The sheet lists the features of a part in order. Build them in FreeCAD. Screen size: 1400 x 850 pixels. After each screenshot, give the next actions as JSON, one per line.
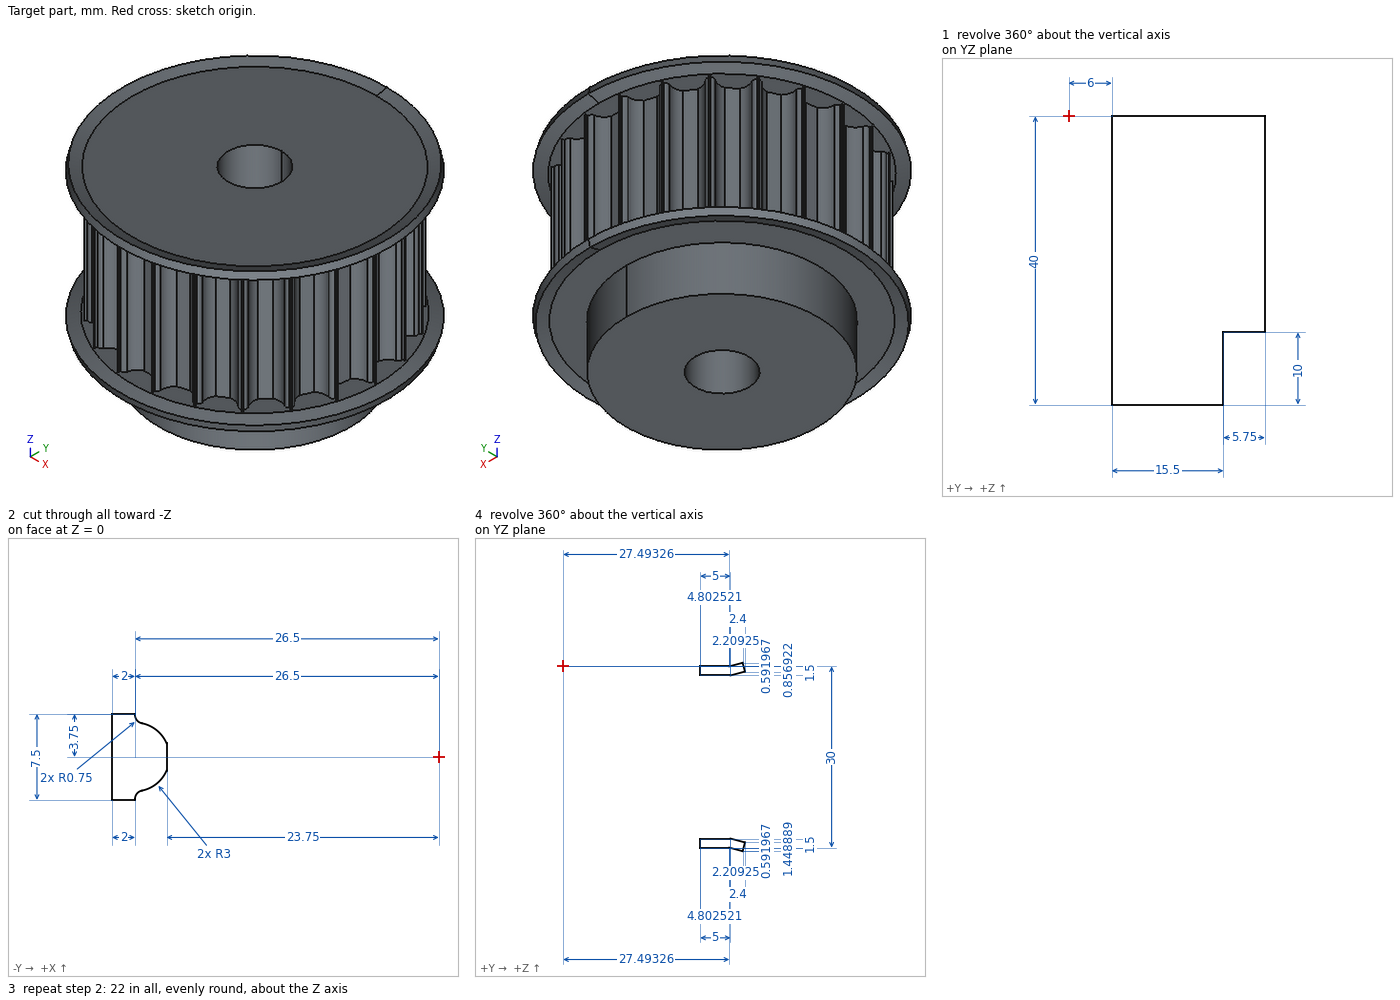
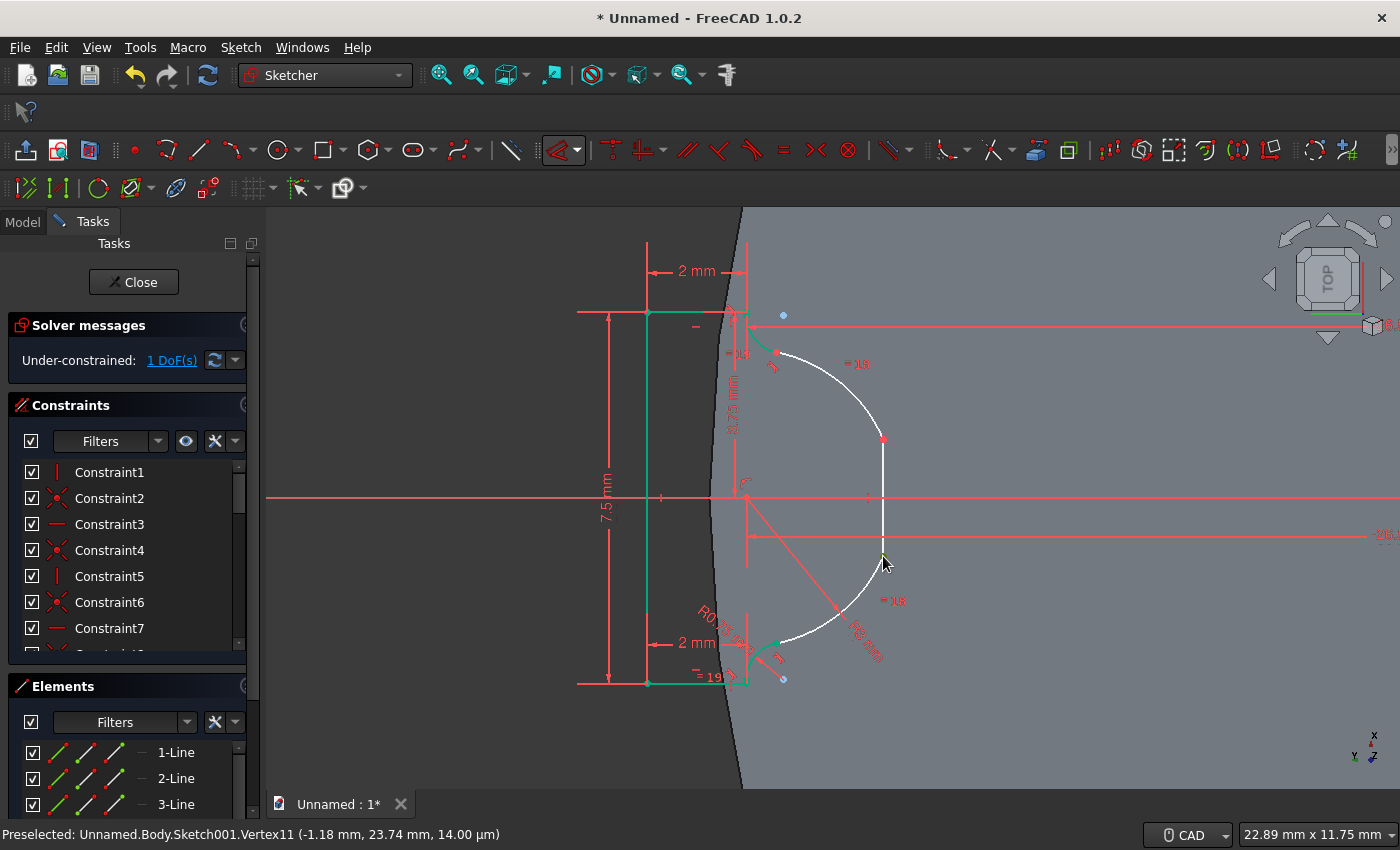
{"action": "key", "text": "l"}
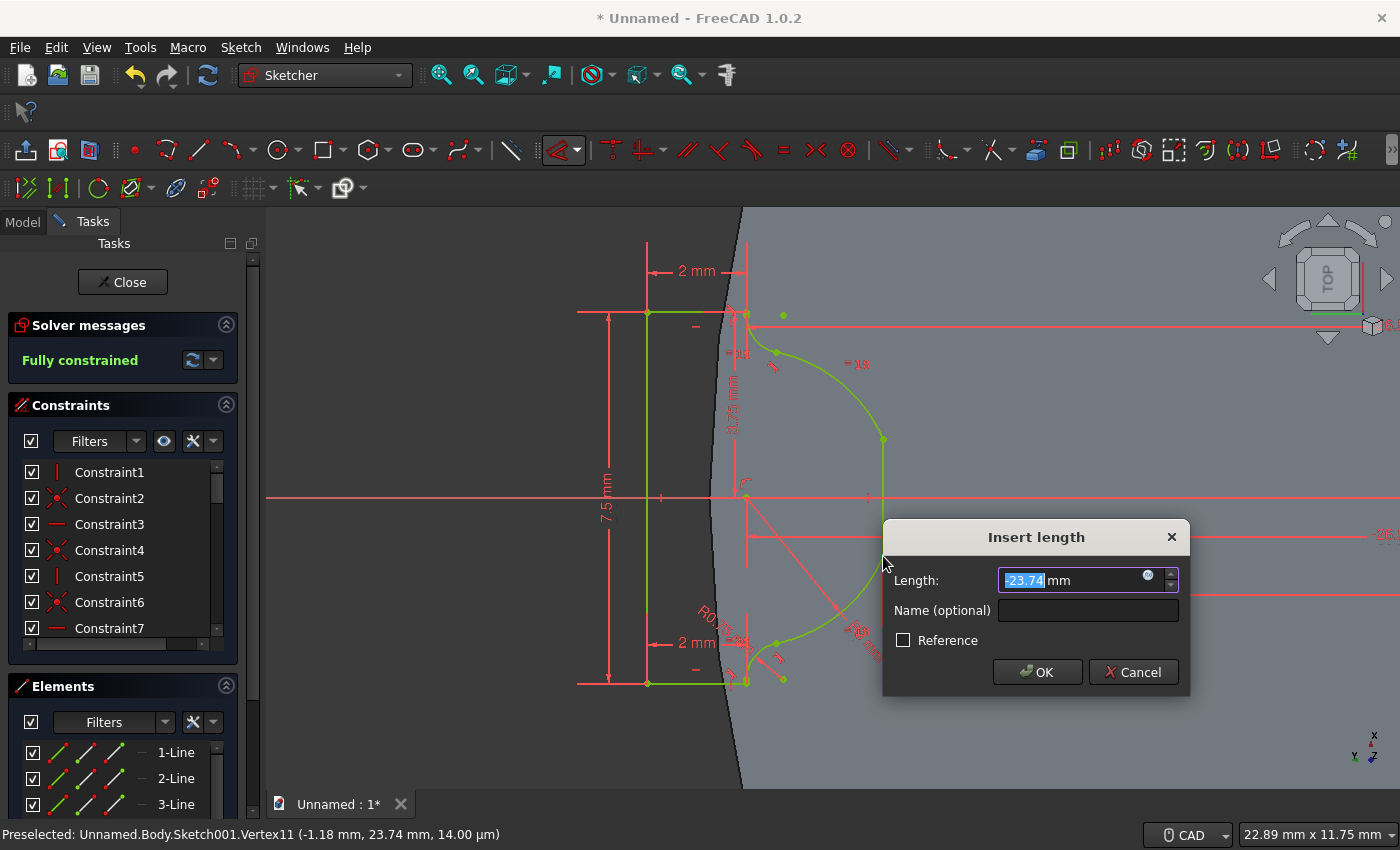
{"action": "type", "text": "-23.75"}
{"action": "key", "text": "Return"}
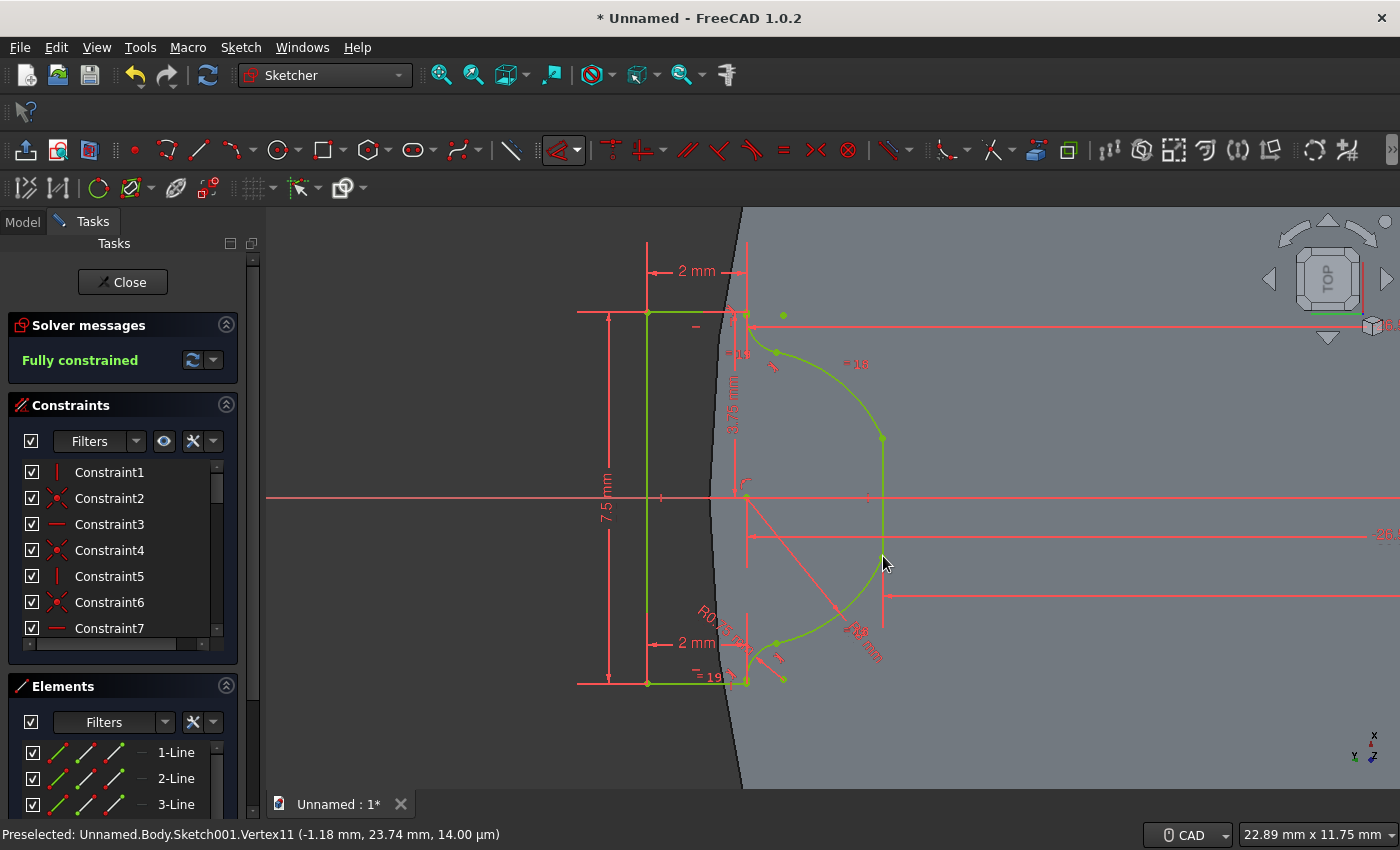
{"action": "left_click", "coordinate": [123, 282]}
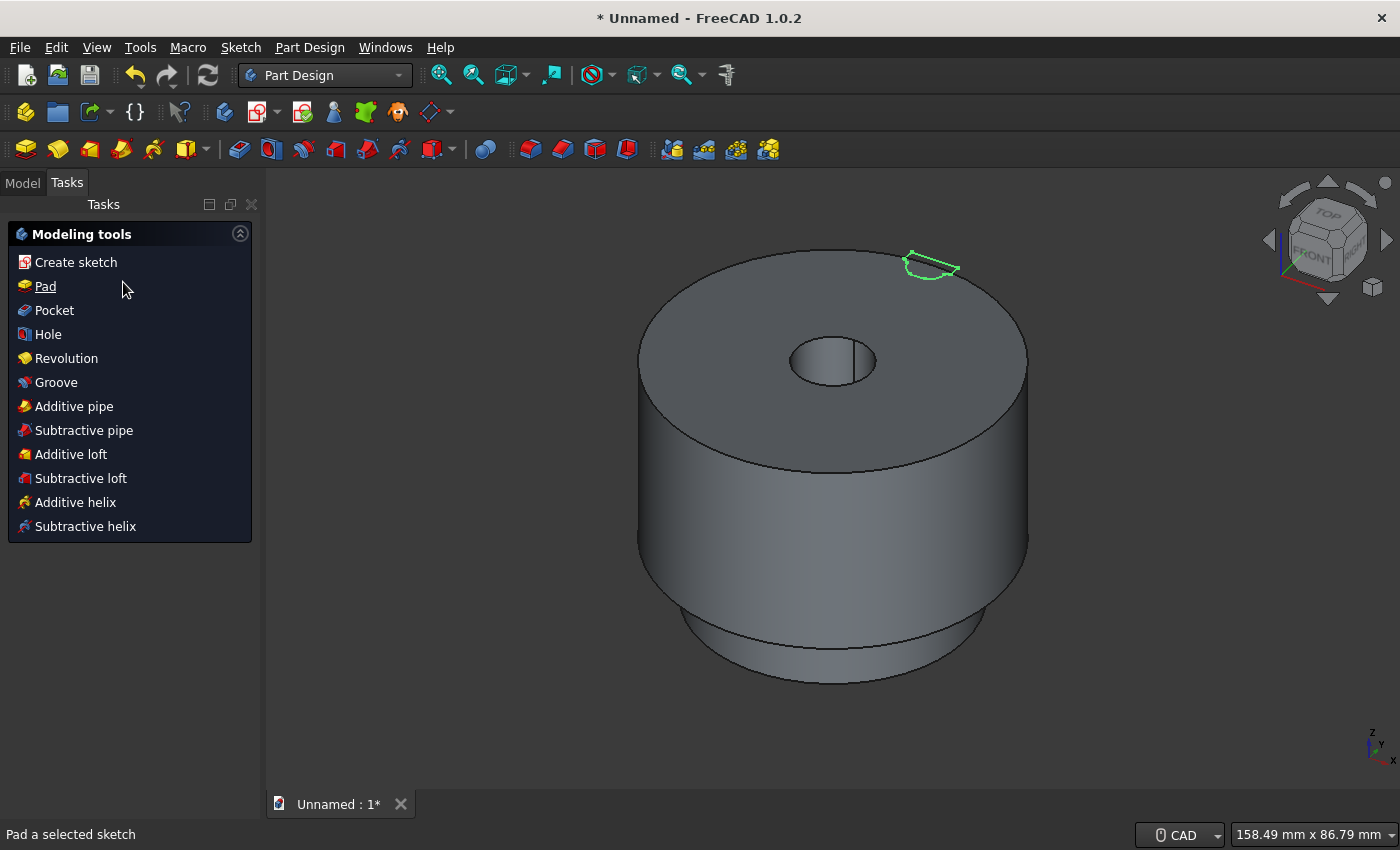
{"action": "left_click", "coordinate": [240, 150]}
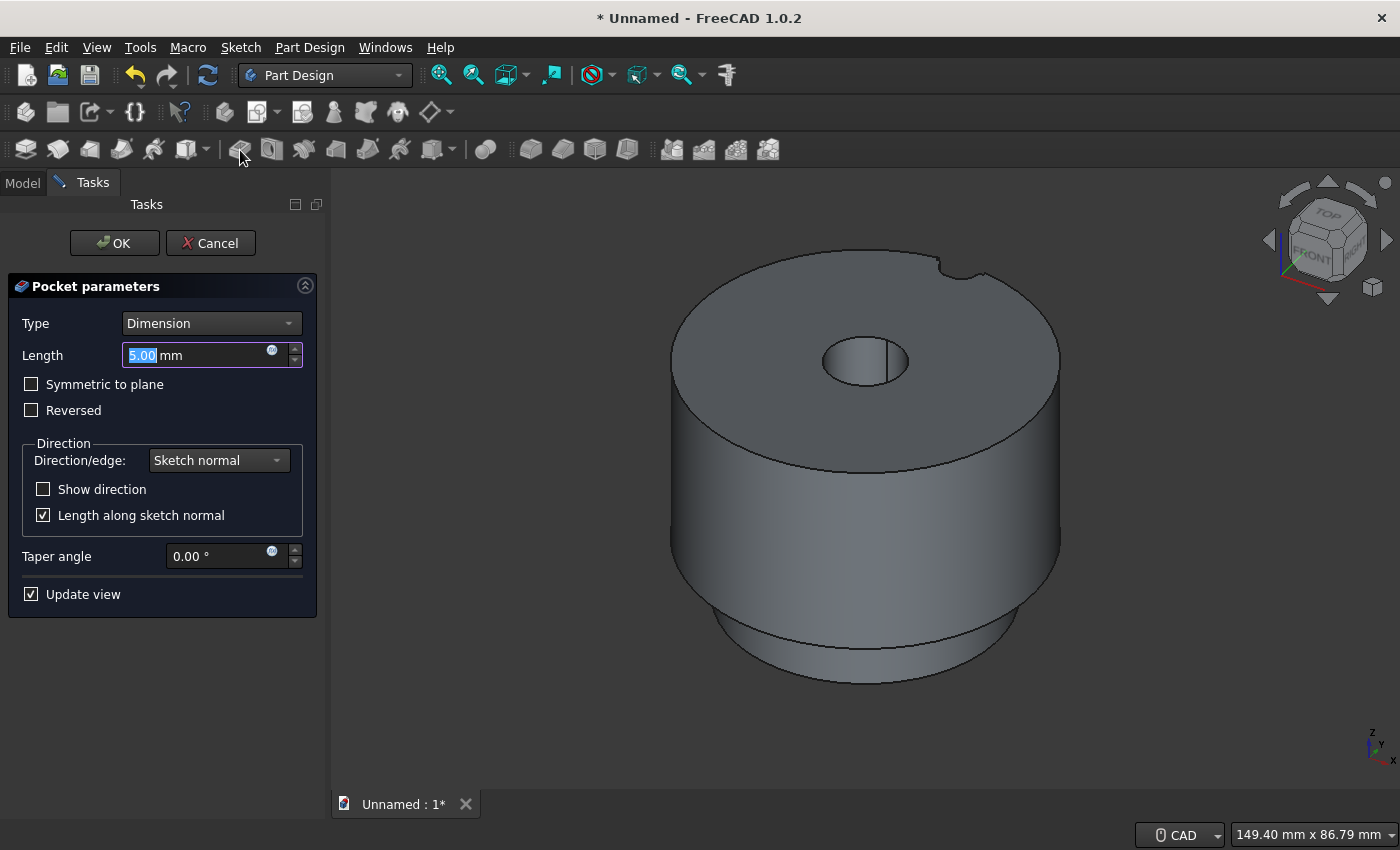
{"action": "left_click", "coordinate": [212, 324]}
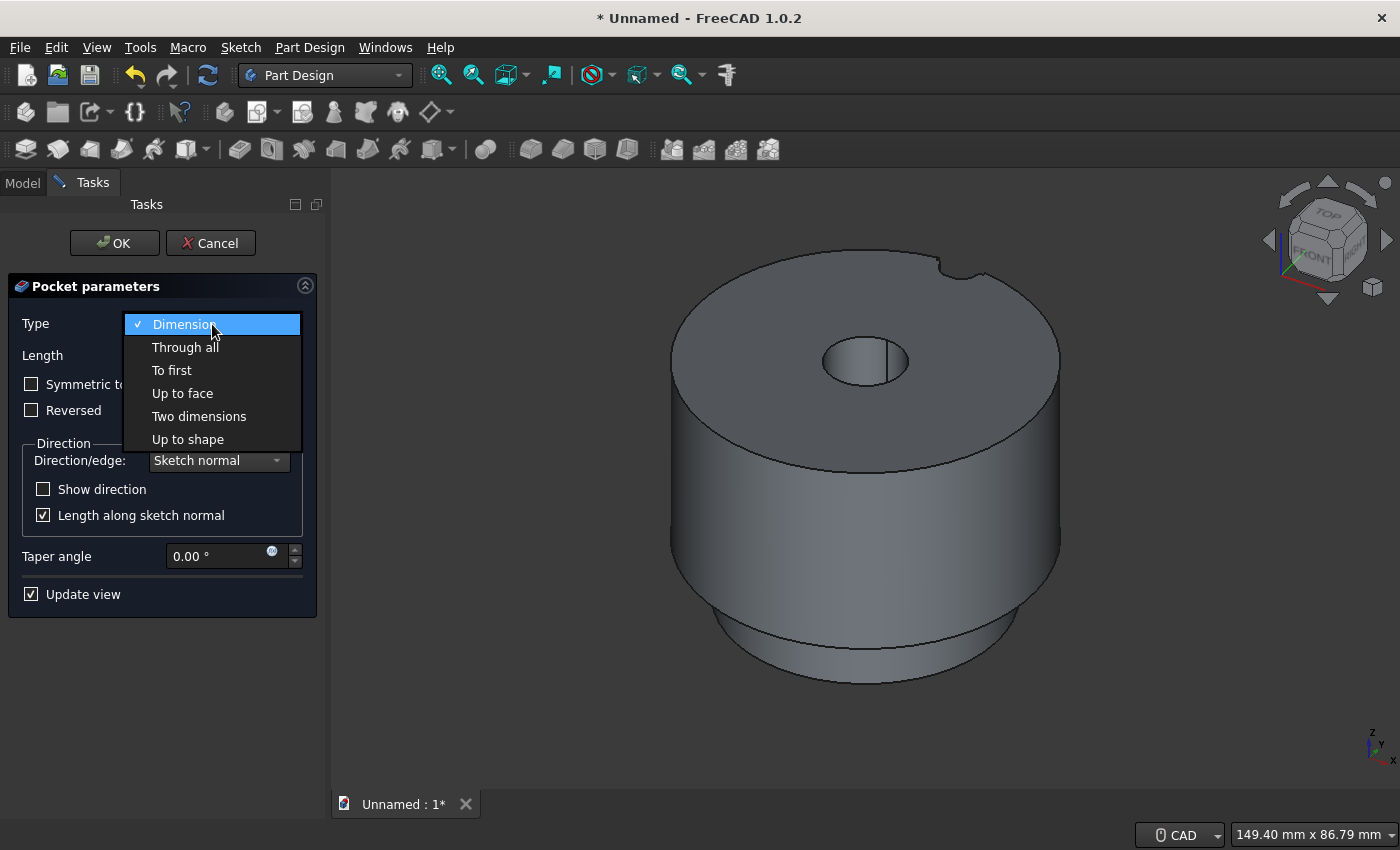
{"action": "left_click", "coordinate": [212, 348]}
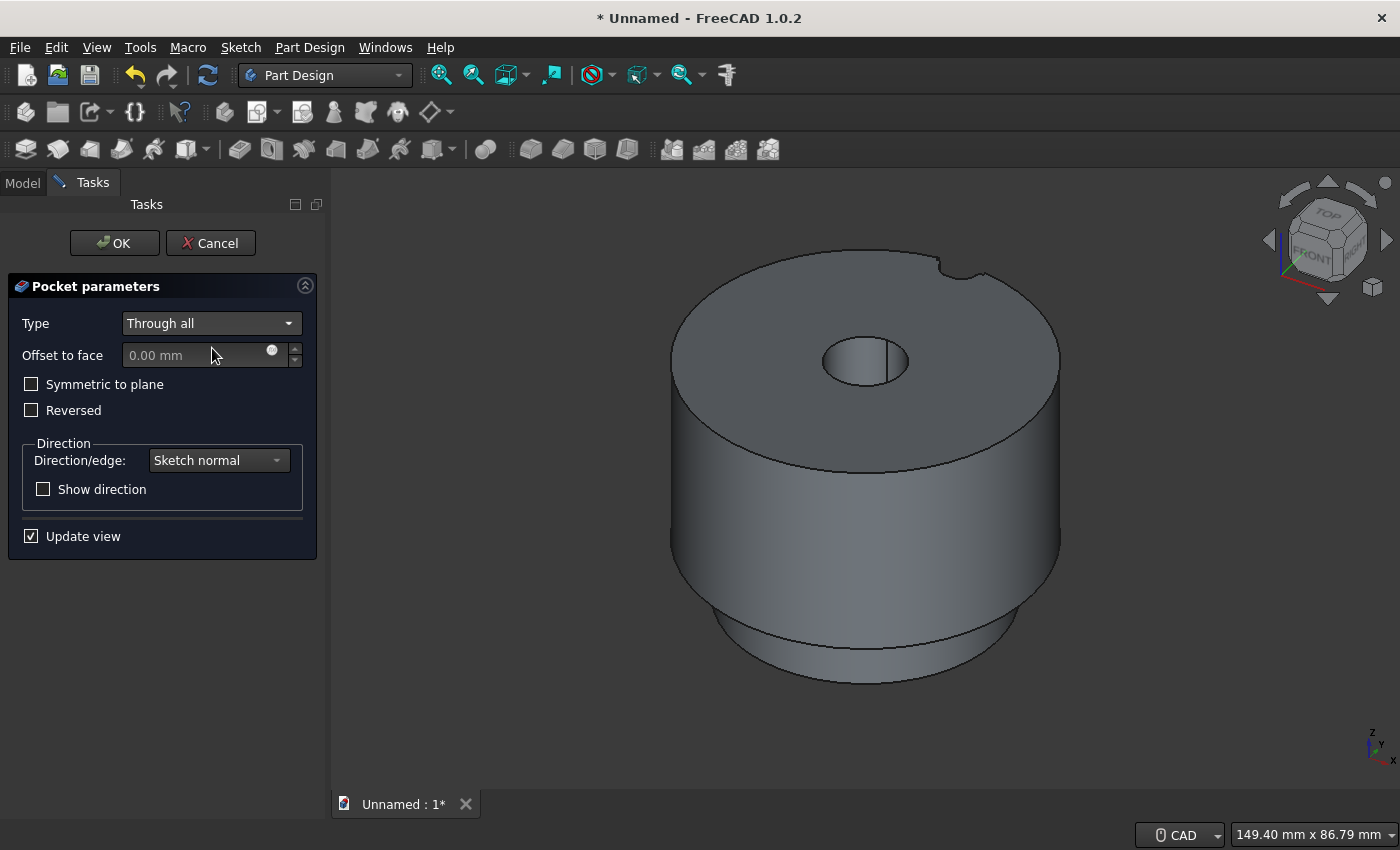
{"action": "left_click", "coordinate": [115, 243]}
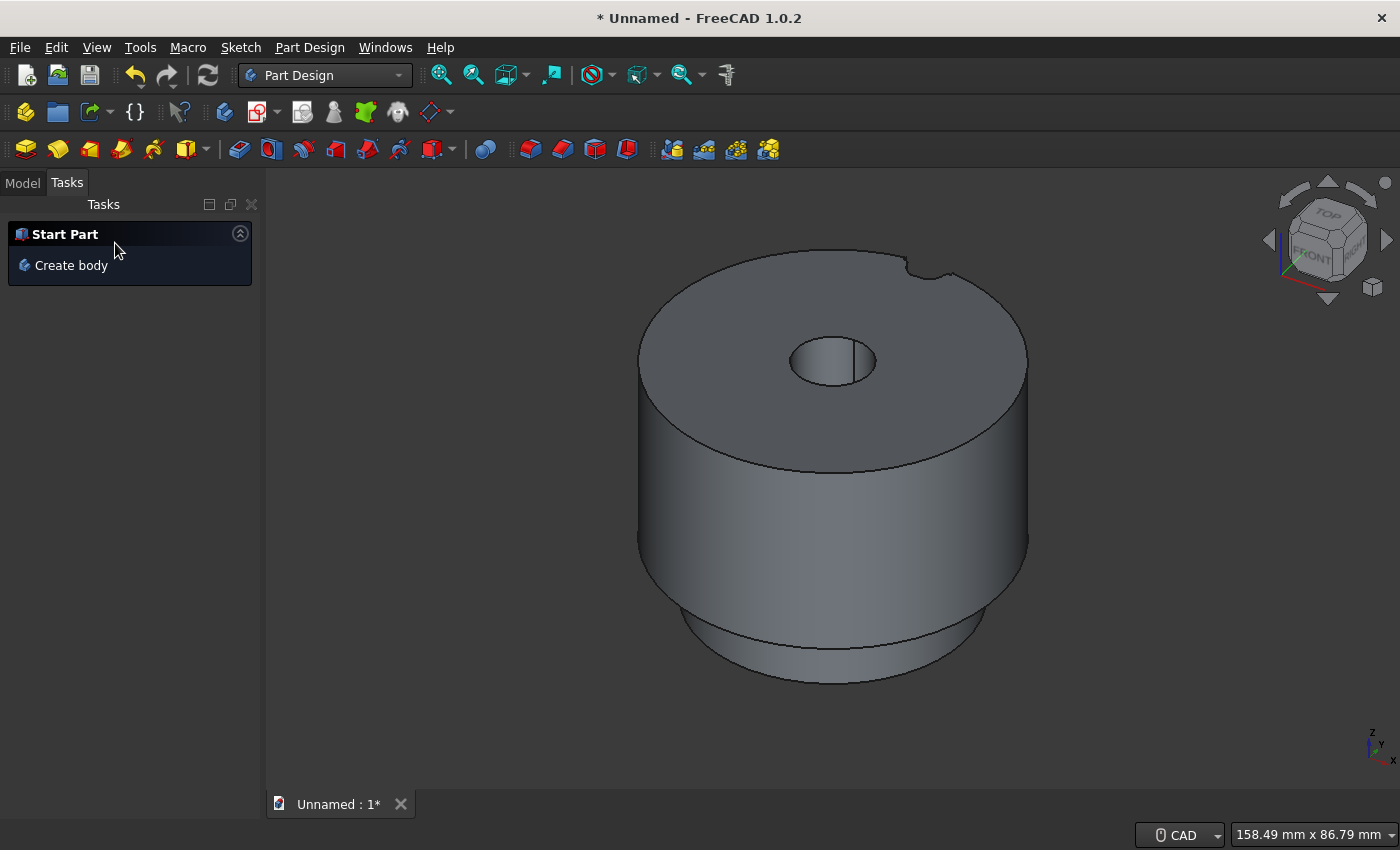
{"action": "left_click", "coordinate": [23, 182]}